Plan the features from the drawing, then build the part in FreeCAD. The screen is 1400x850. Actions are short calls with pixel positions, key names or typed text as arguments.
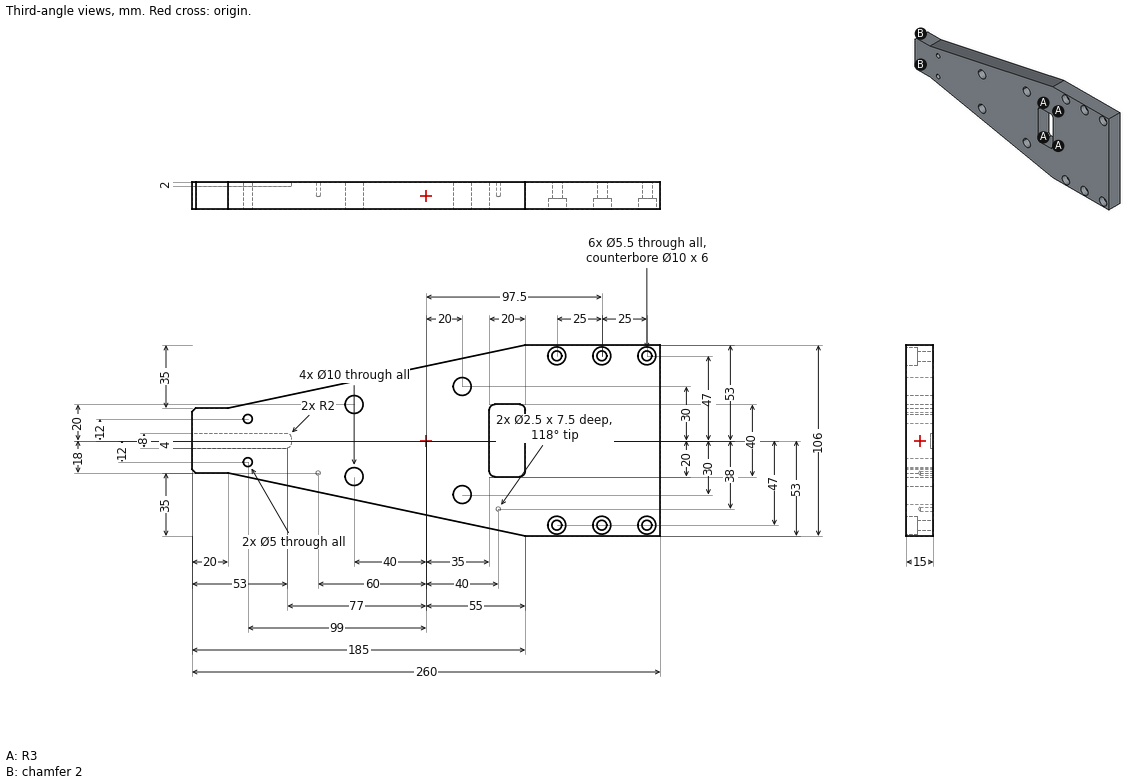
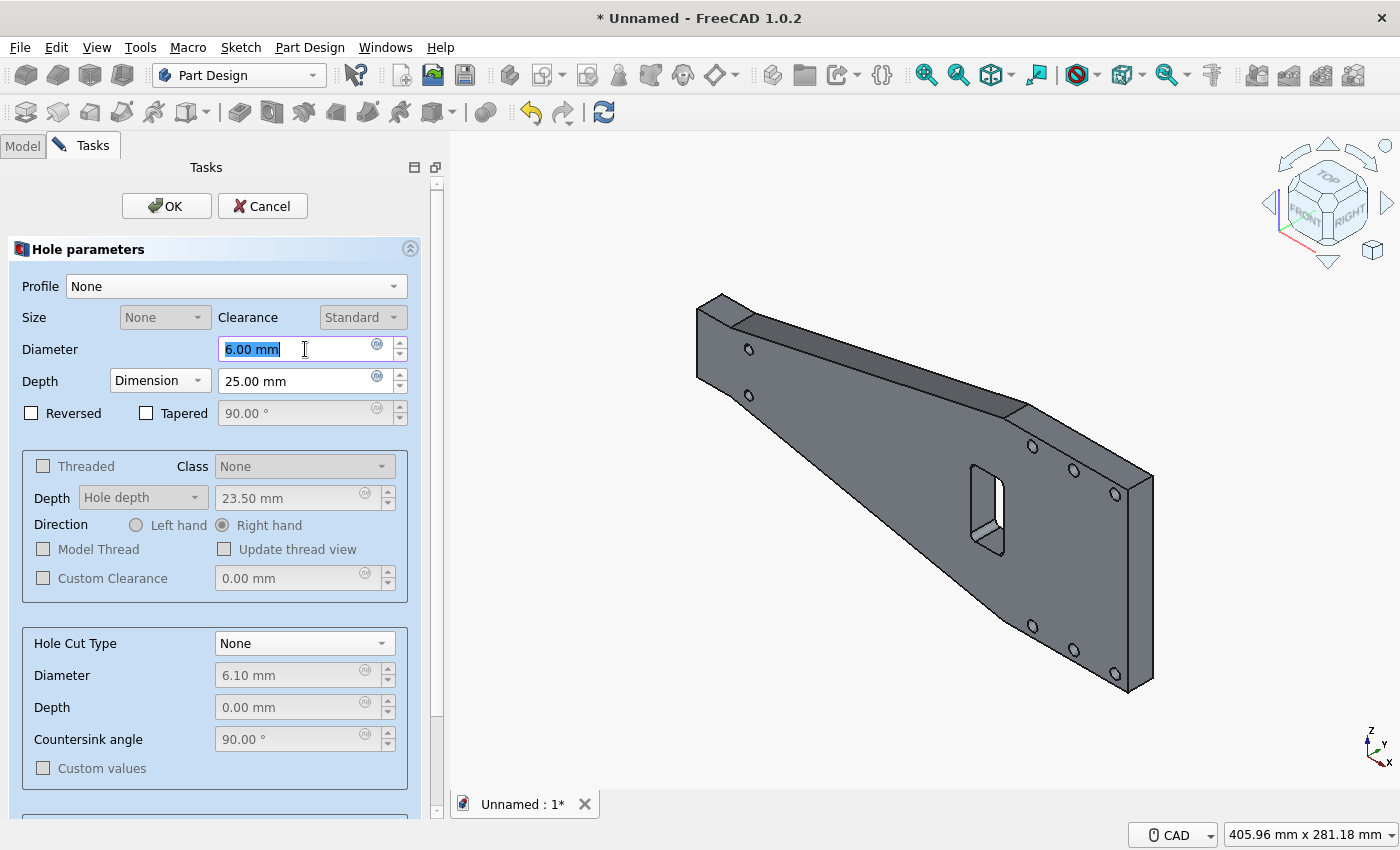
text(5.5)
key(Tab)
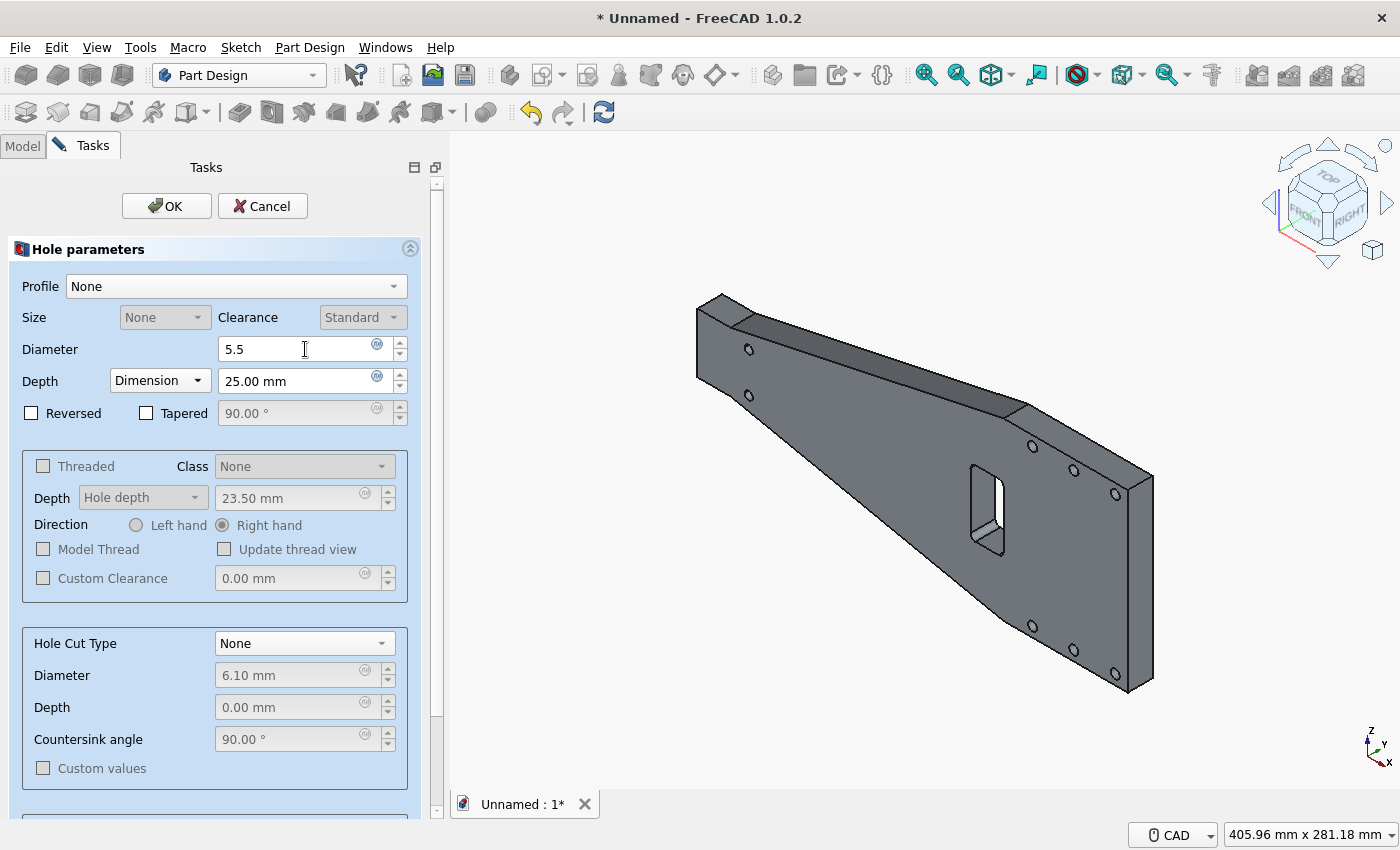
click(161, 380)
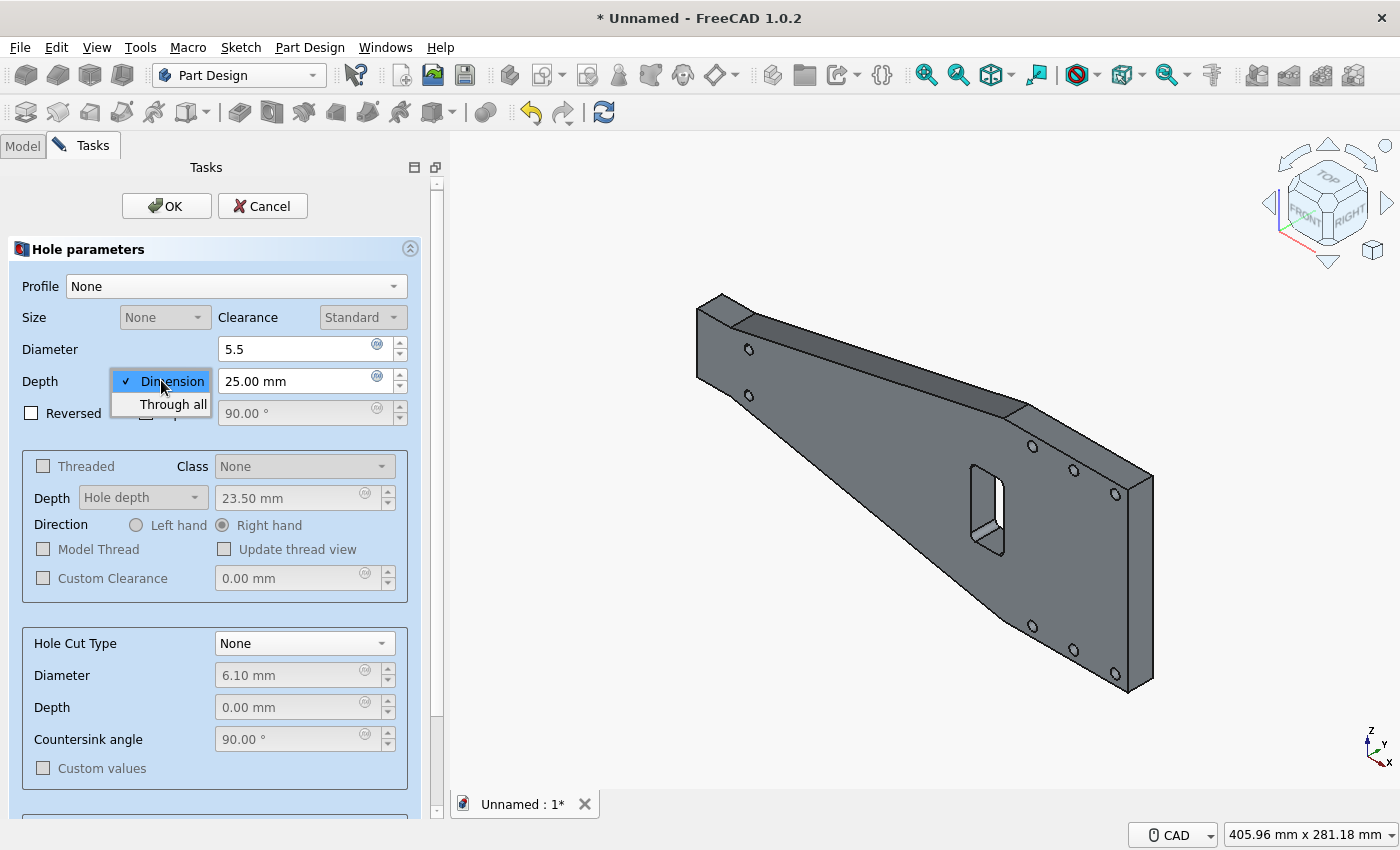
click(160, 404)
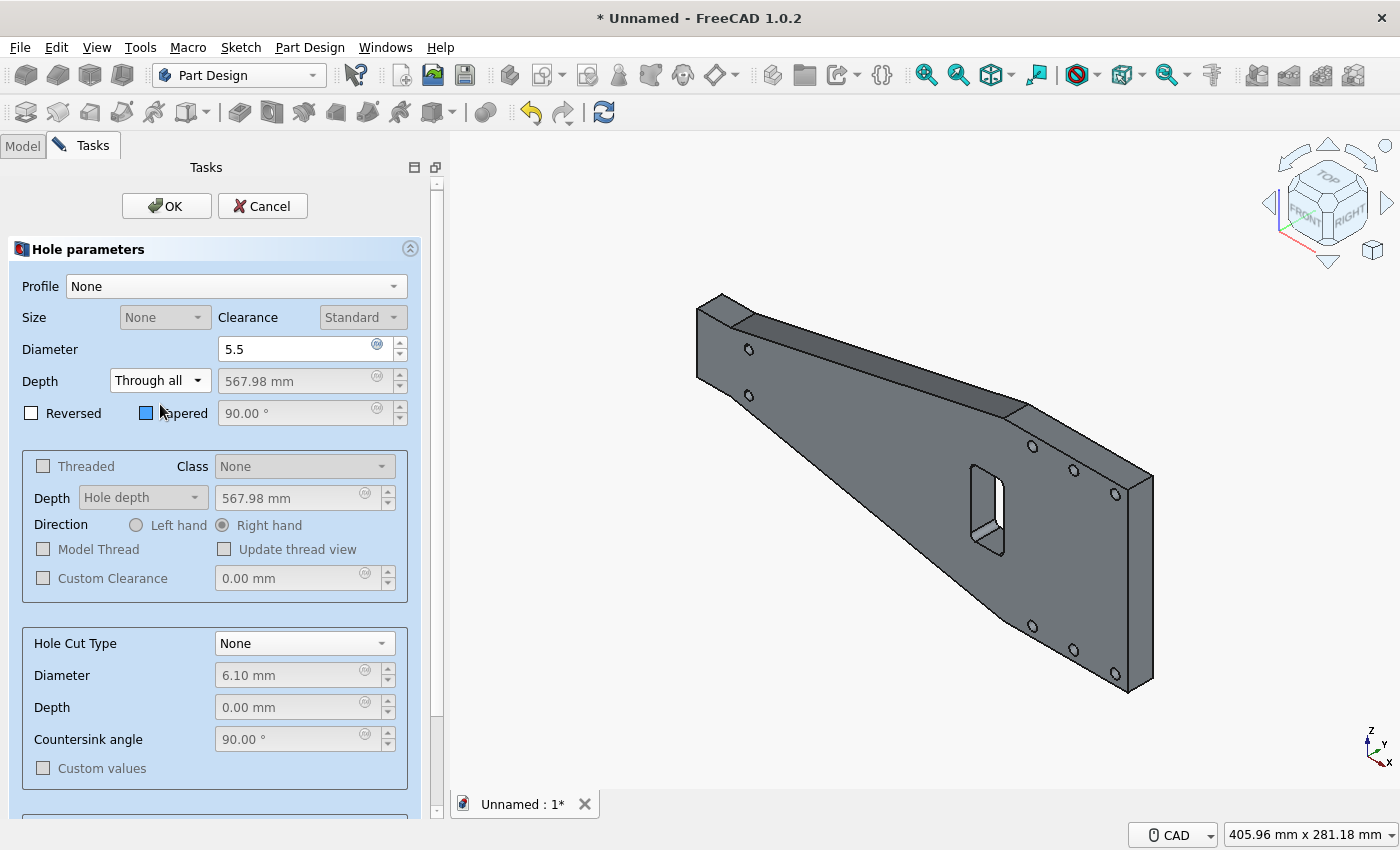
click(306, 644)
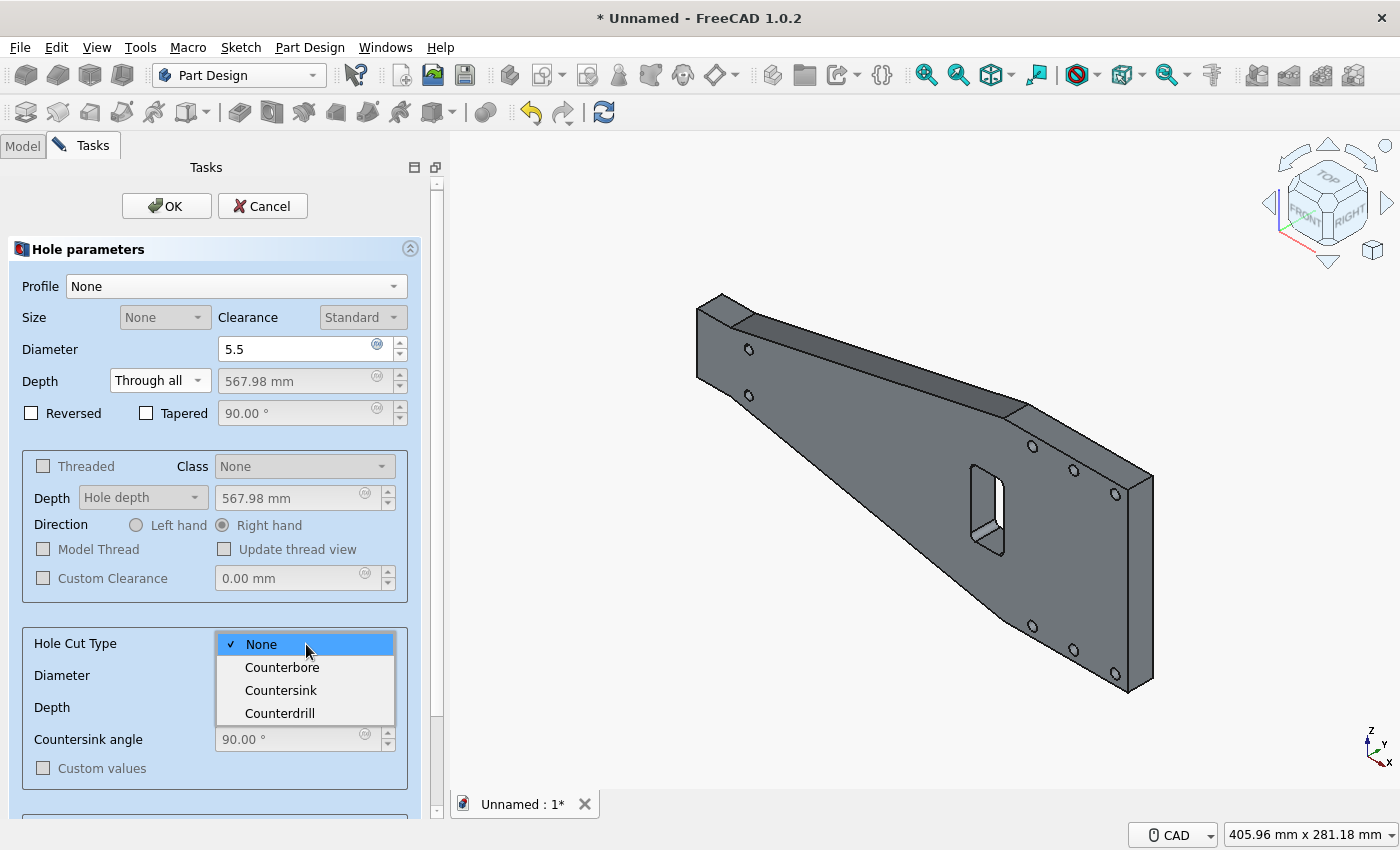
click(304, 668)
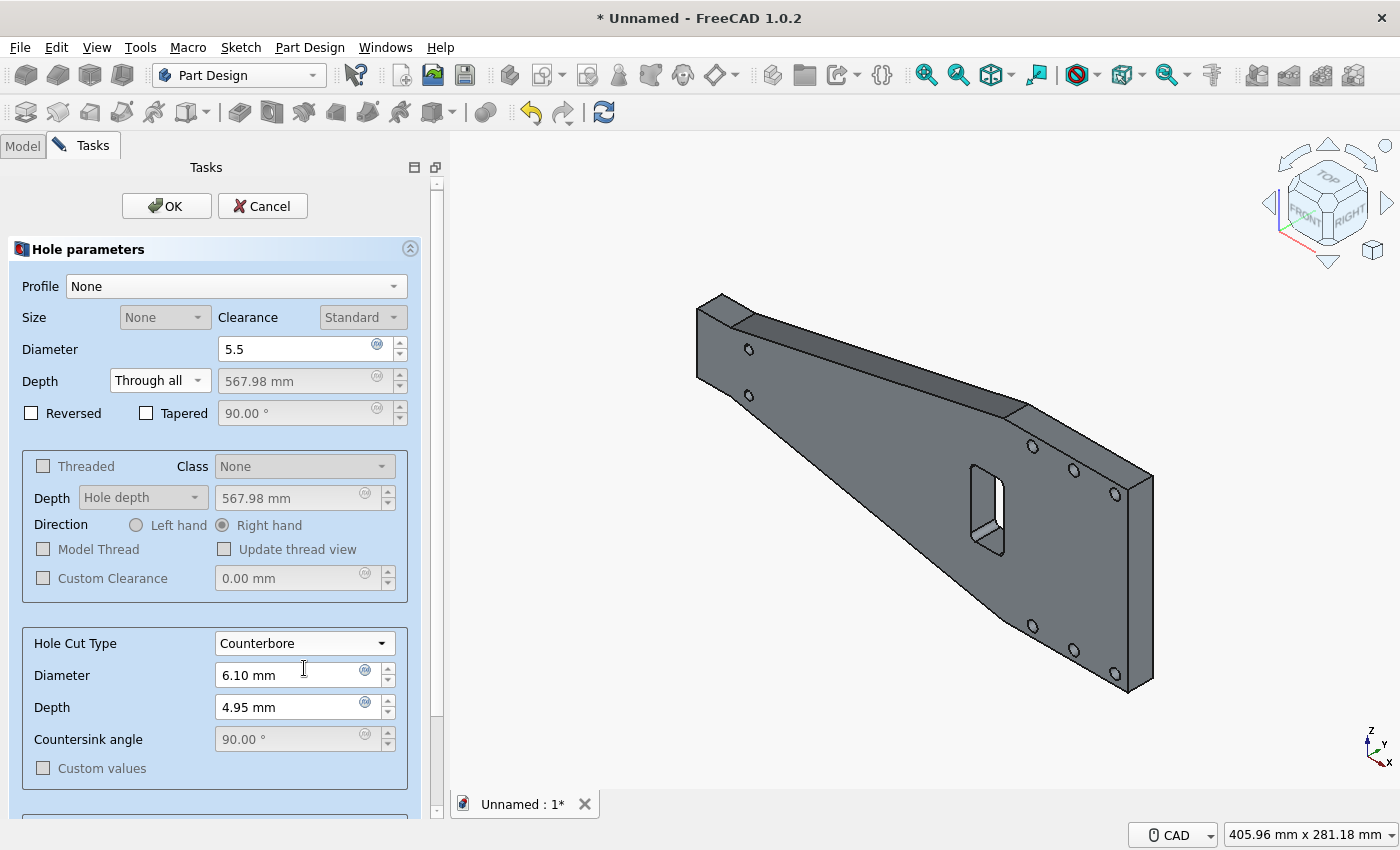
triple_click(298, 675)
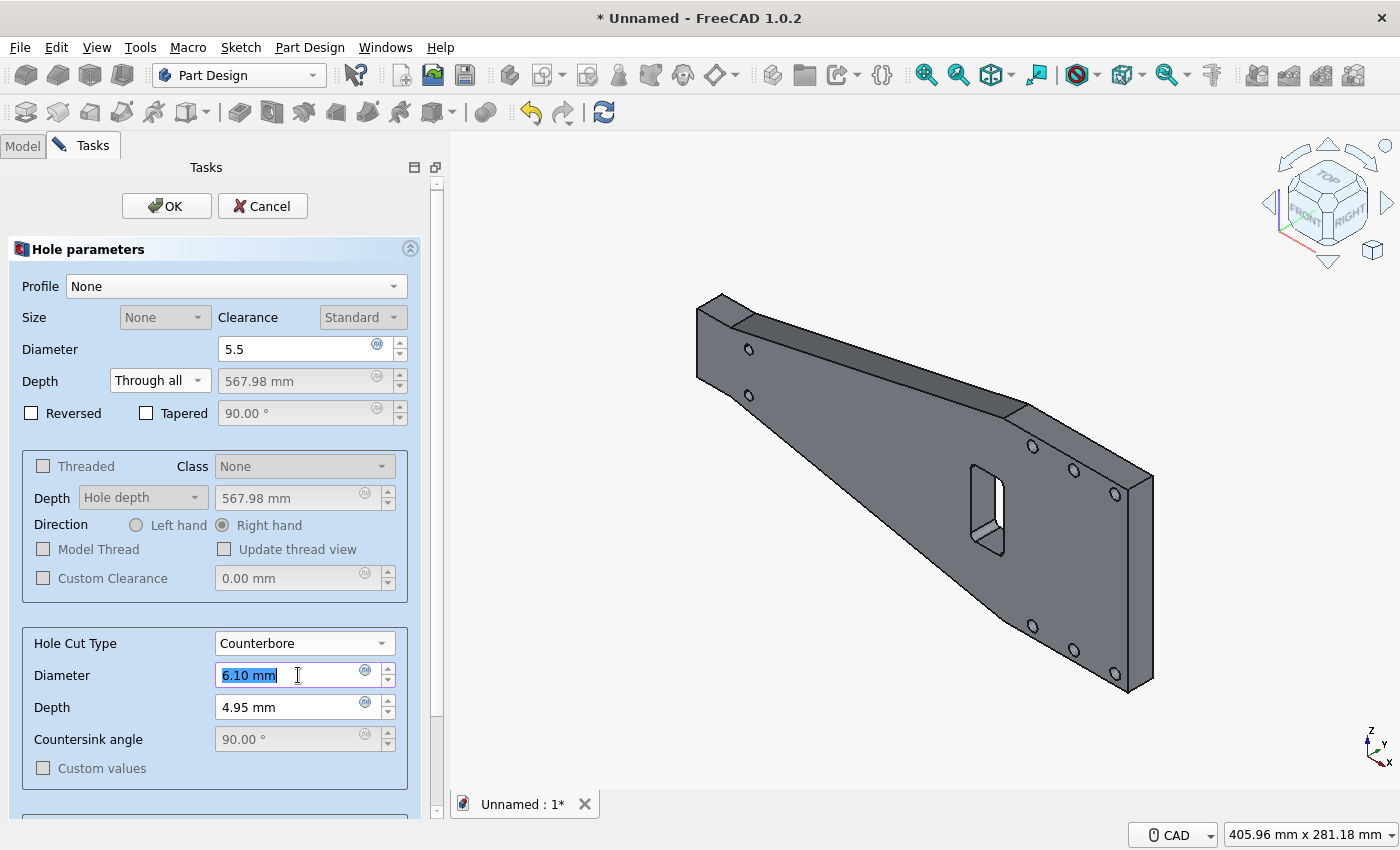
text(10)
key(Tab)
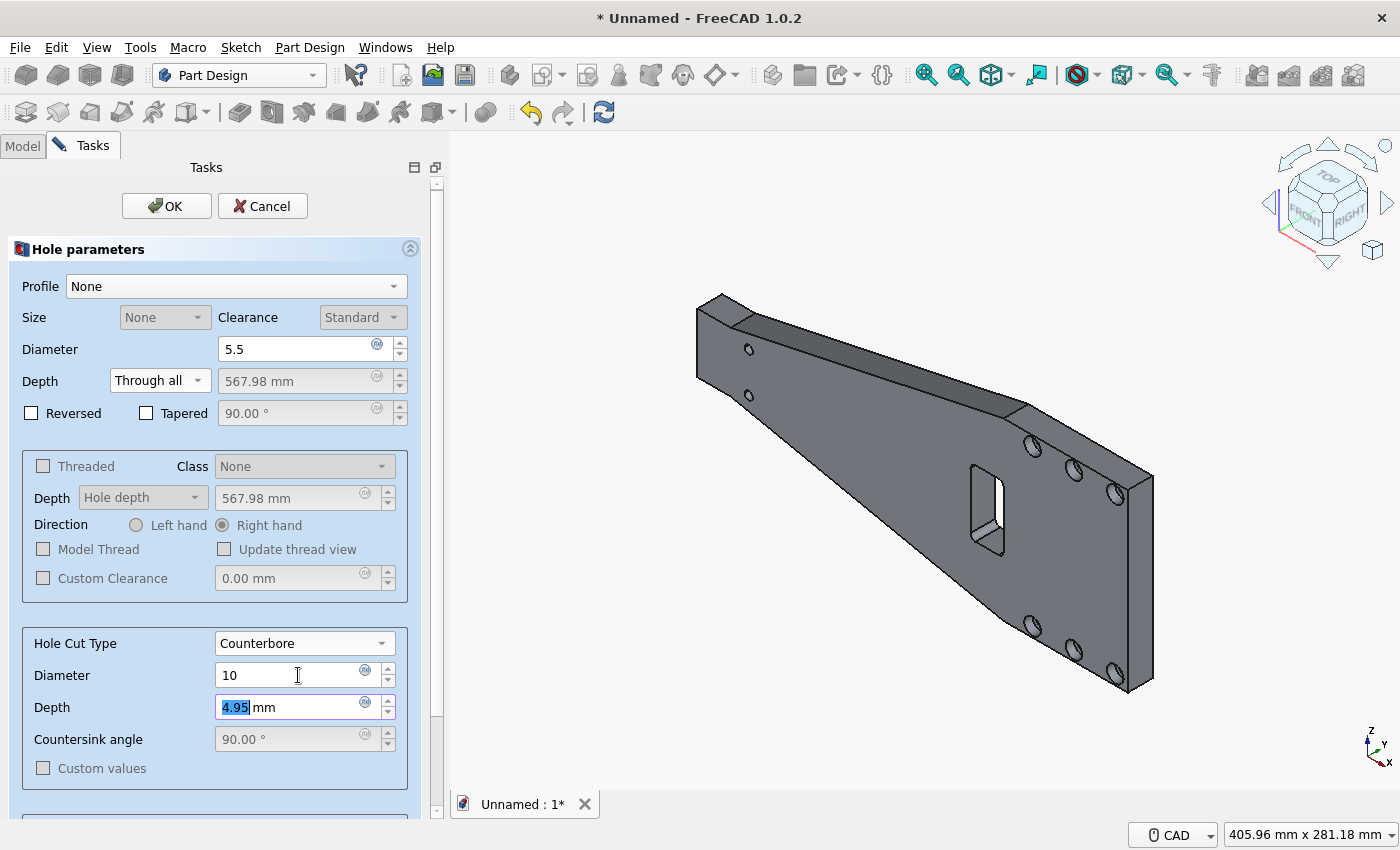
text(6)
key(Tab)